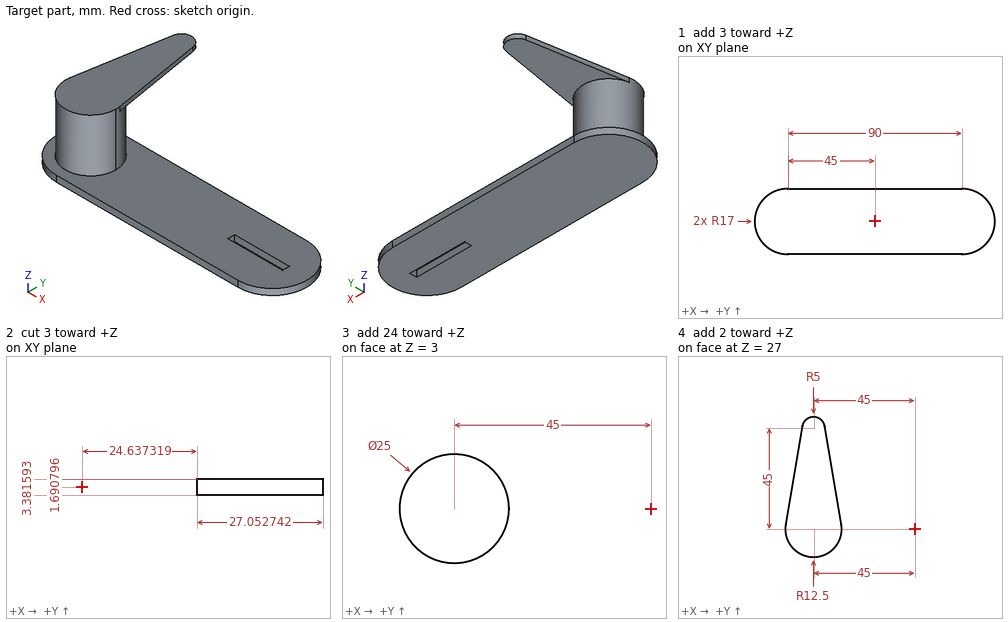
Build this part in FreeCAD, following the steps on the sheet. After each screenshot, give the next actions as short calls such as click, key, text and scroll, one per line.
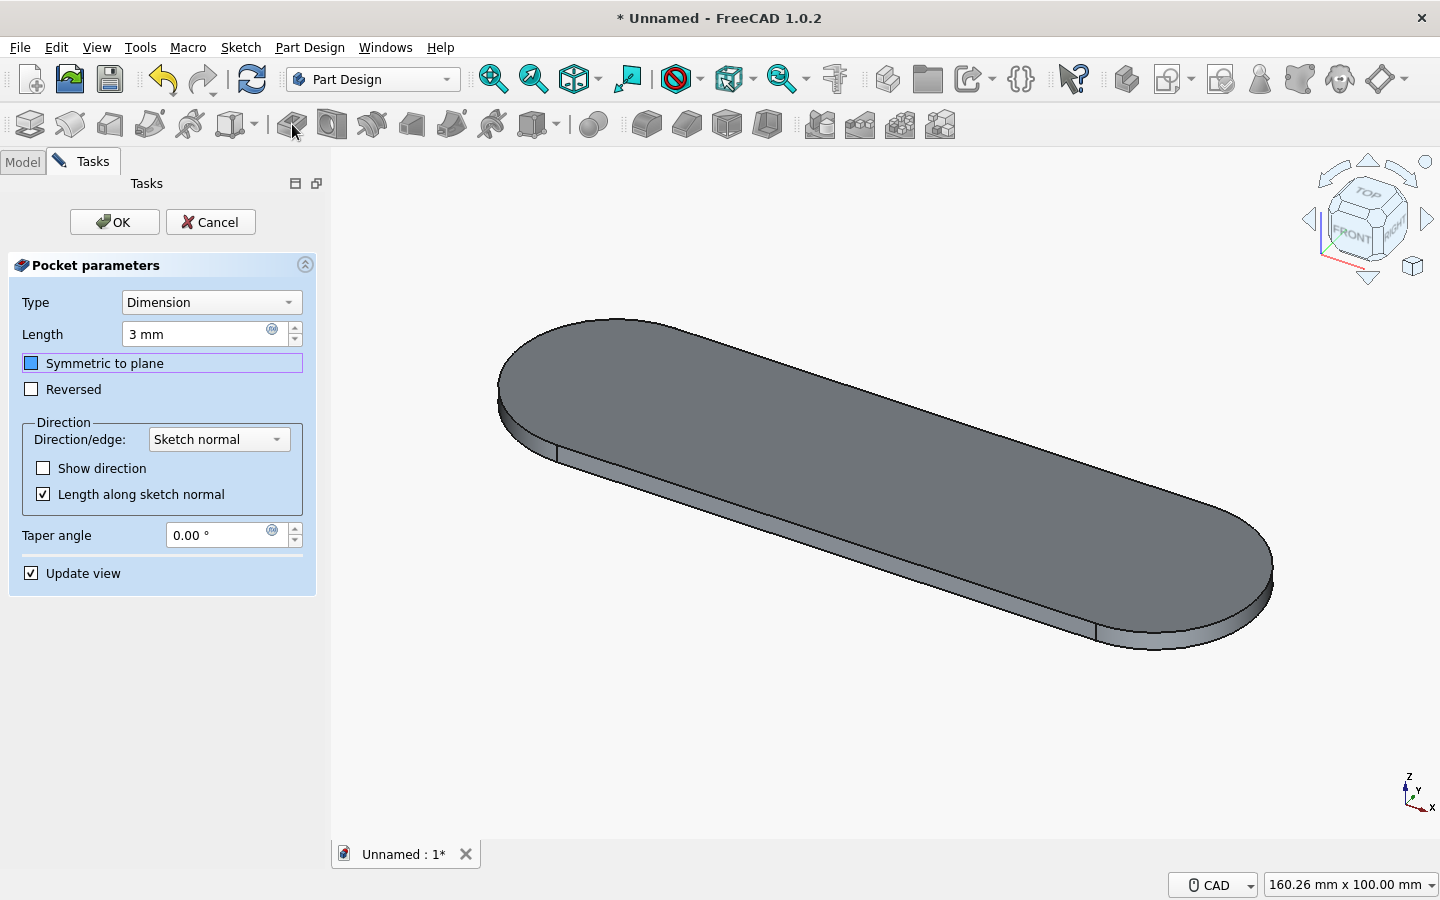
click(30, 389)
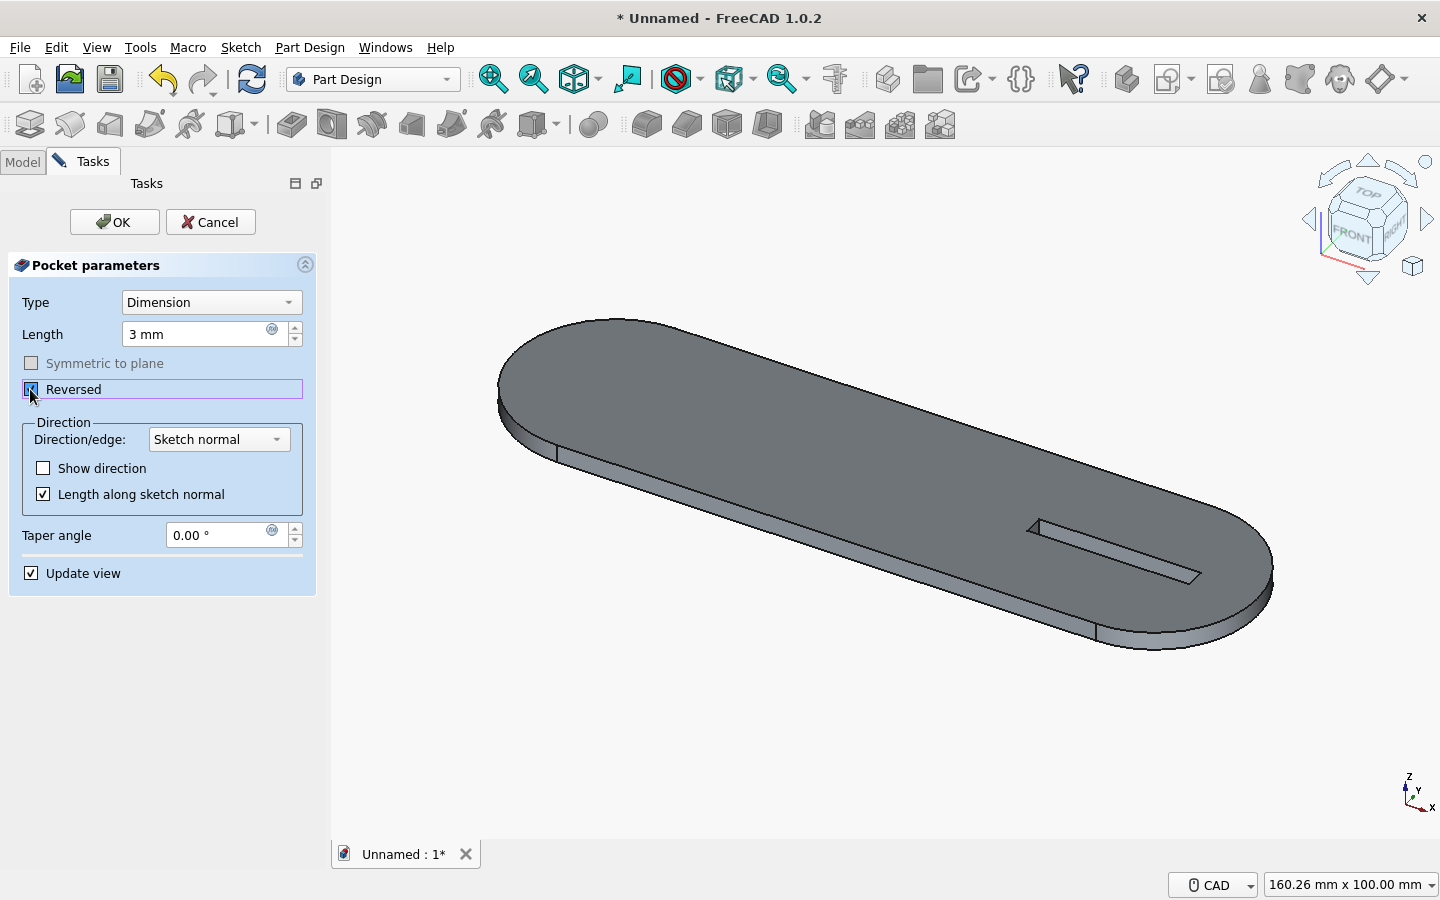
click(115, 222)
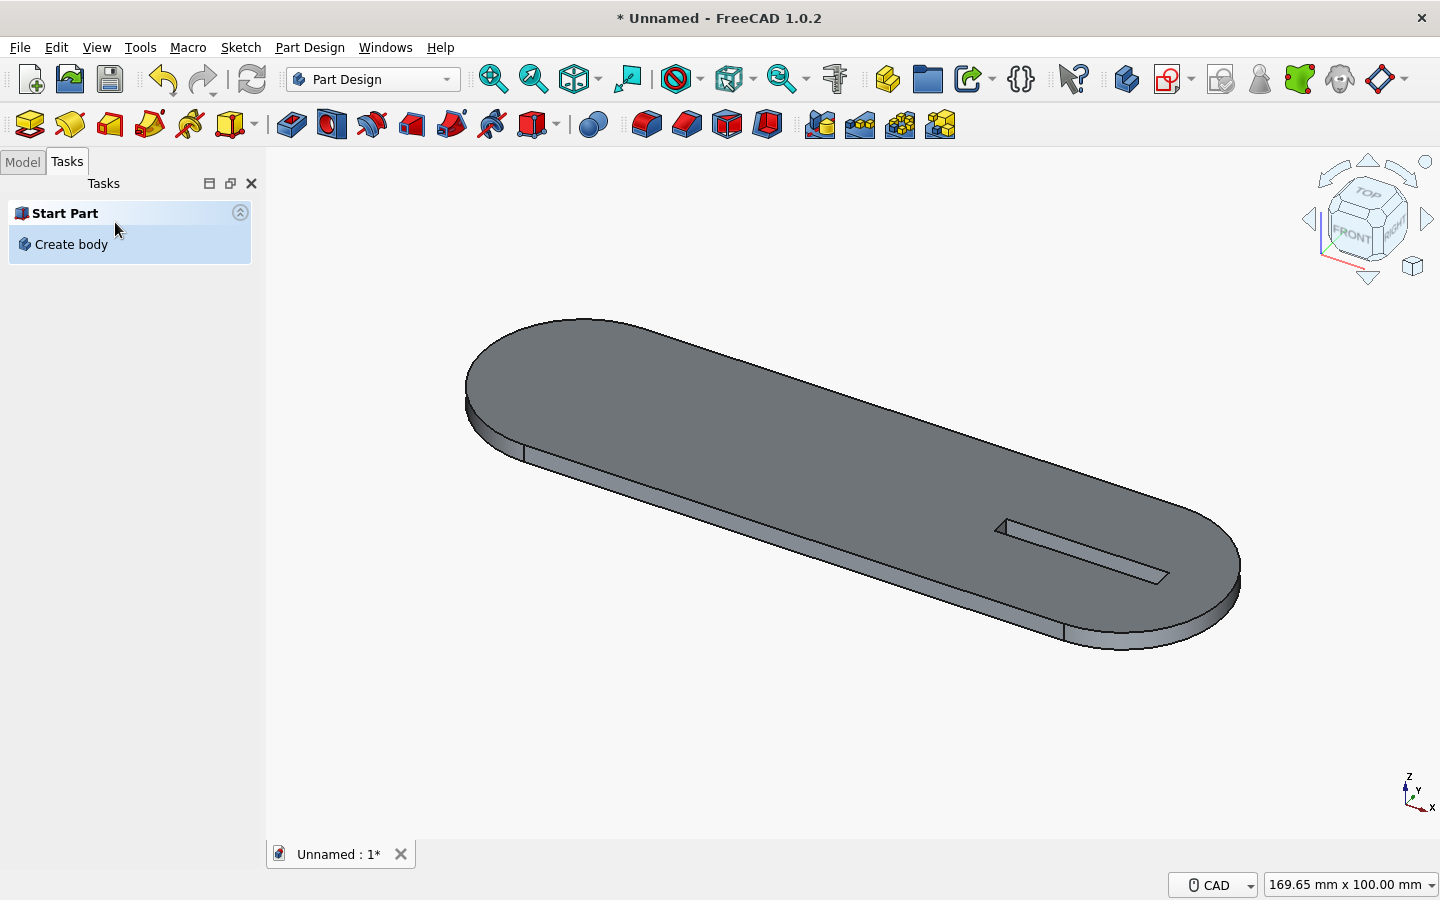
click(853, 475)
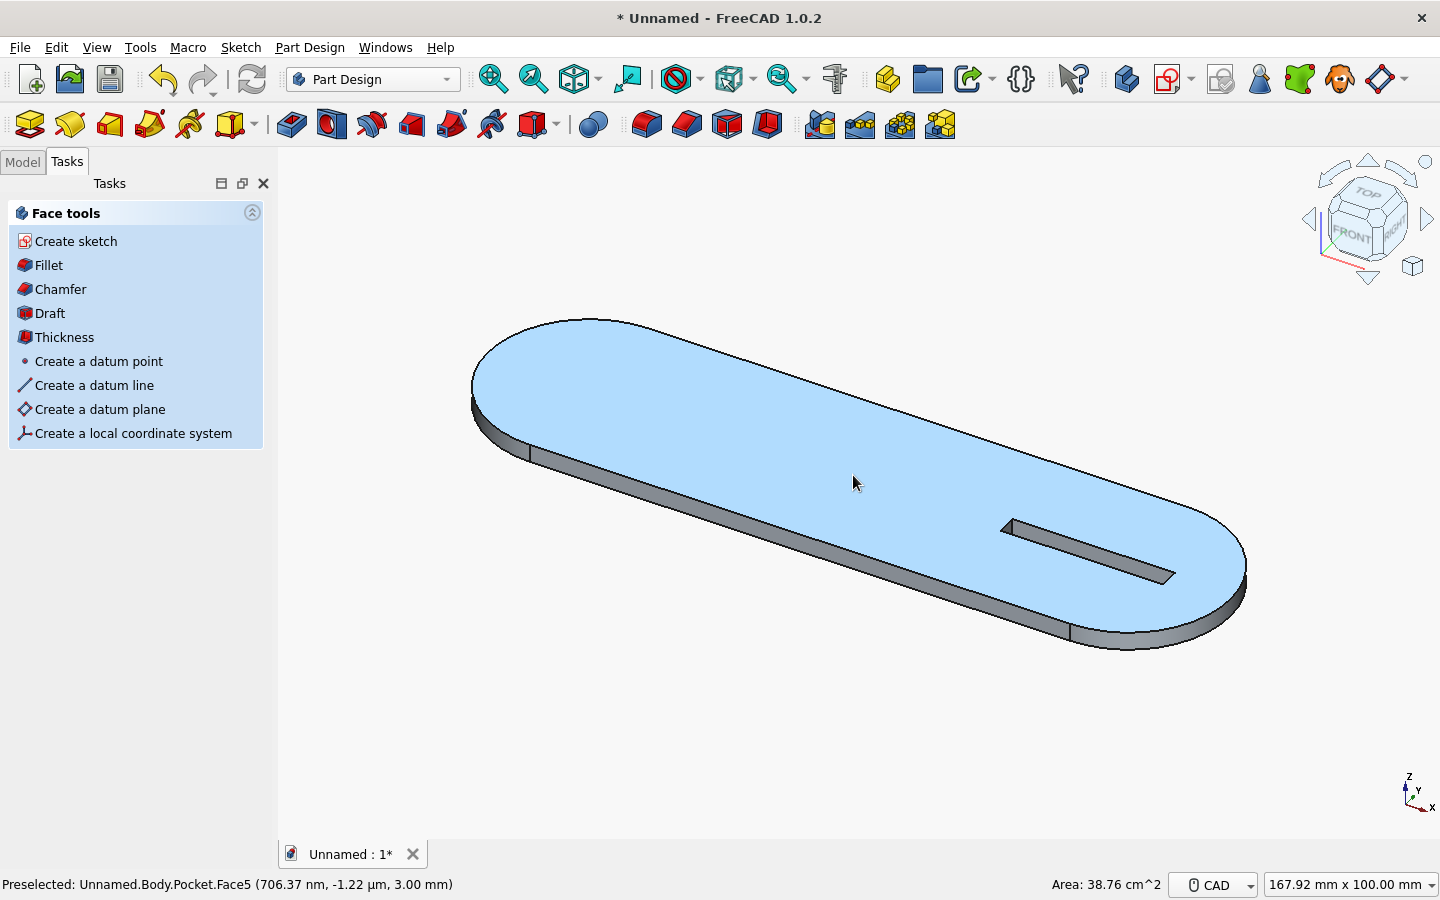
click(1168, 80)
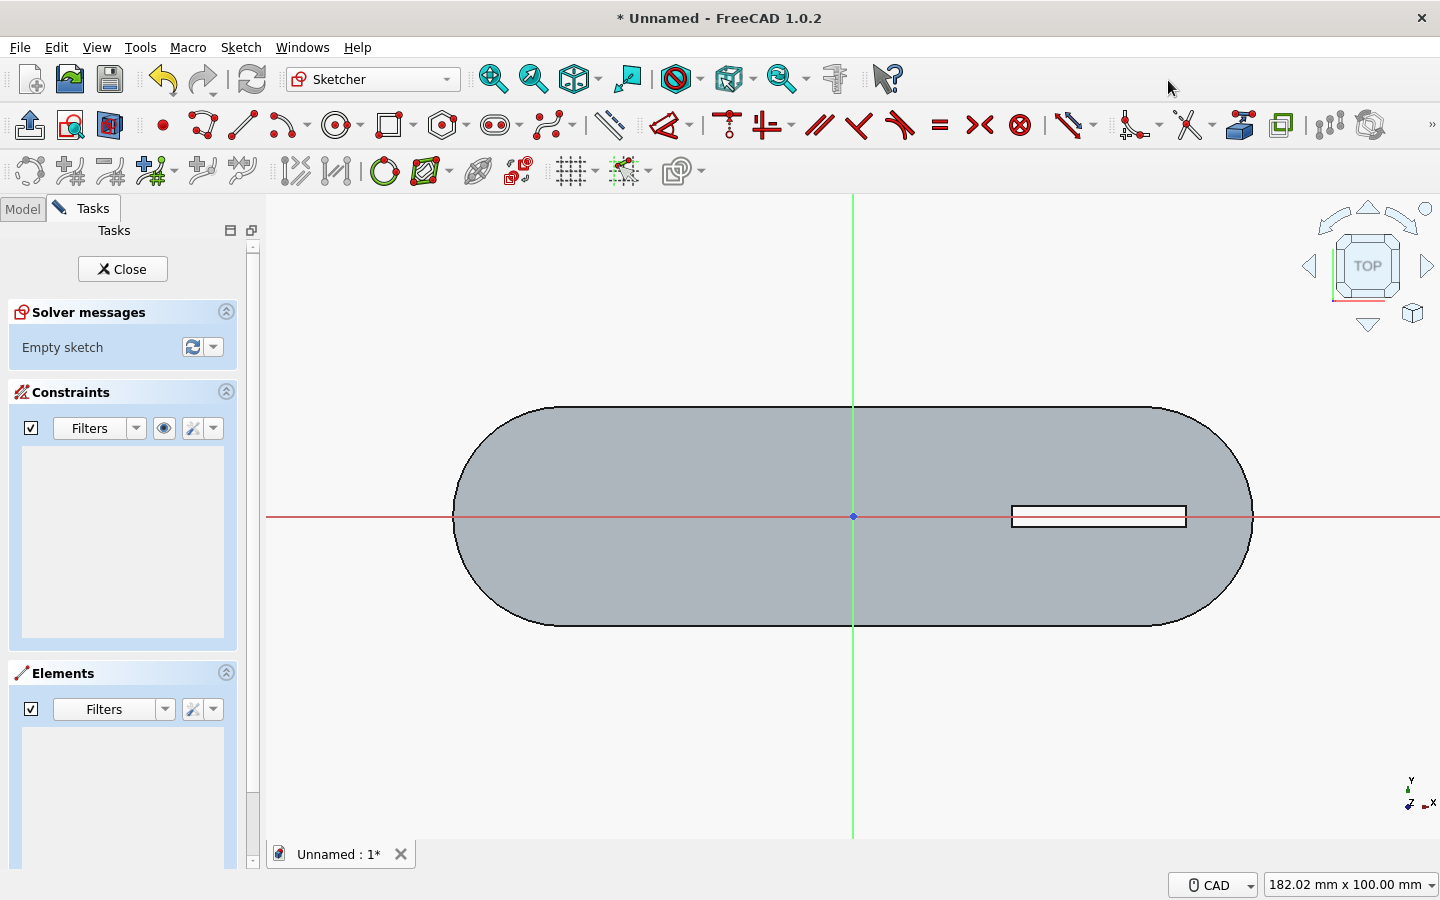
scroll(525, 516, up, 3)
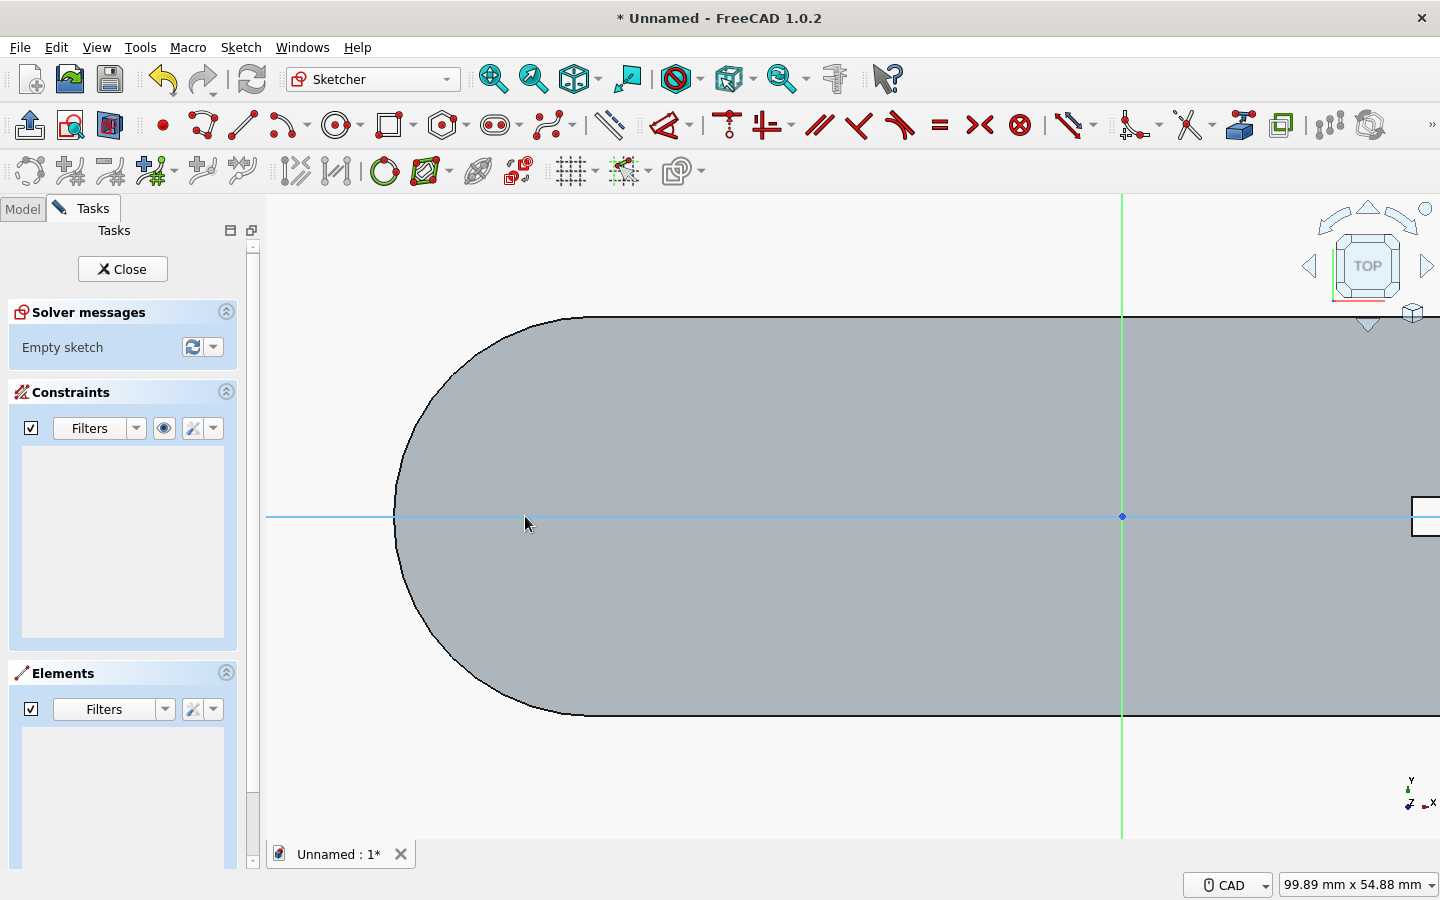
click(336, 126)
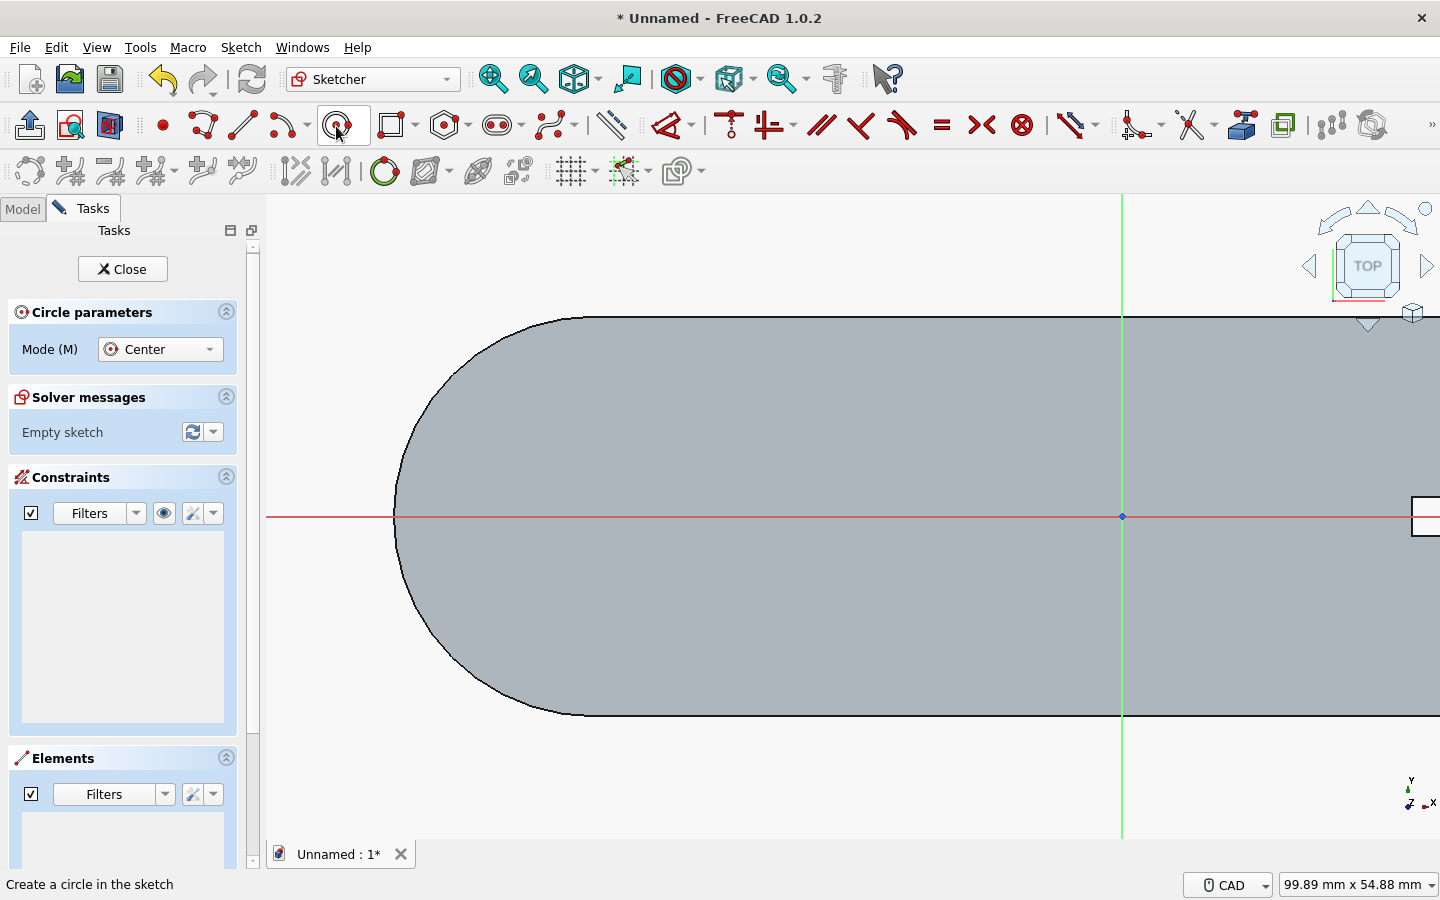
click(594, 516)
click(697, 413)
key(Escape)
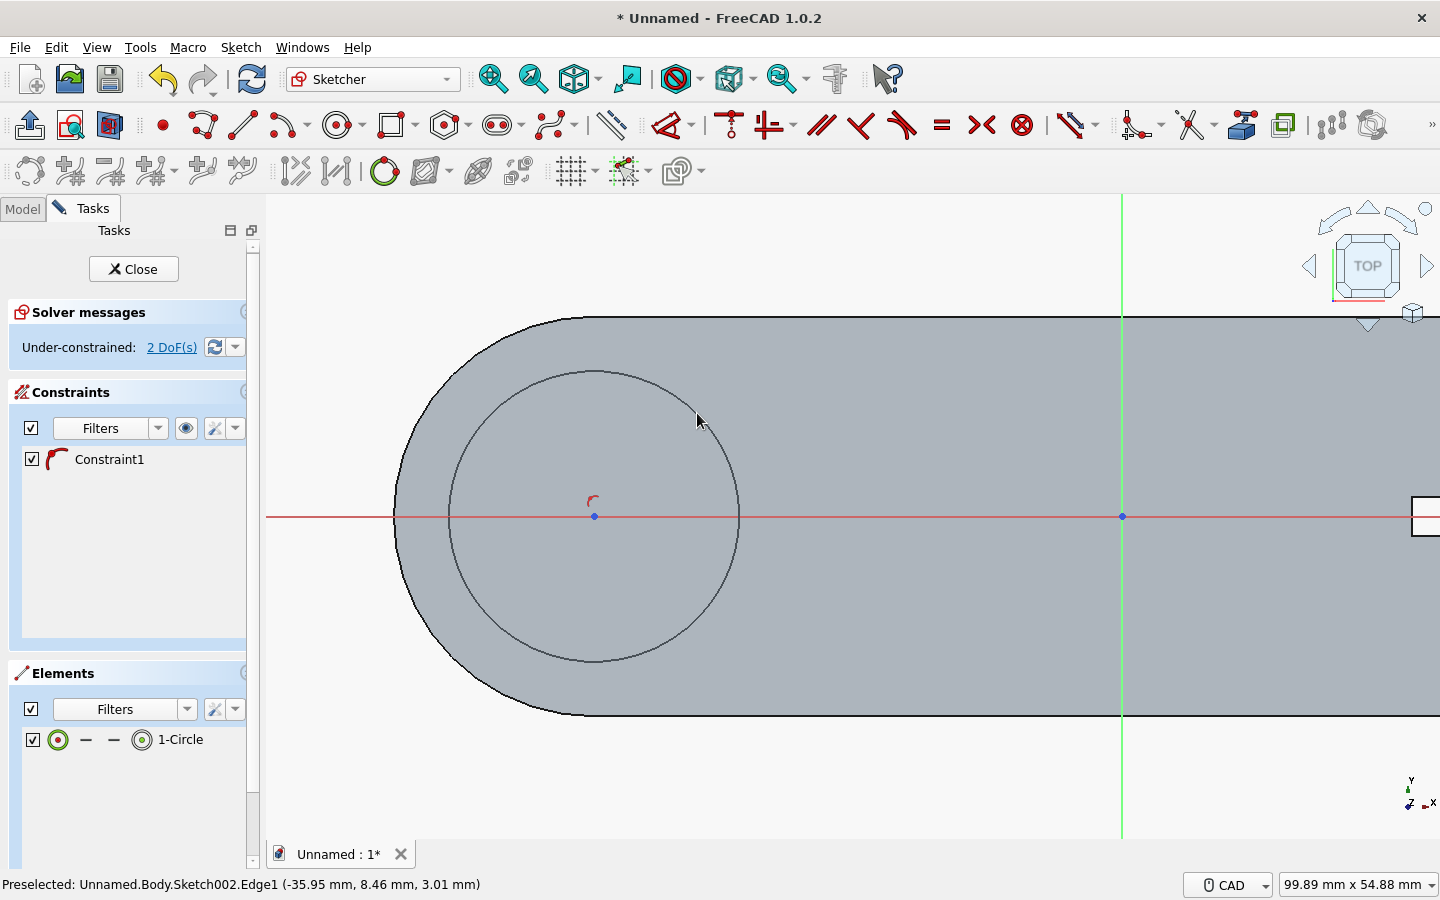
key(d)